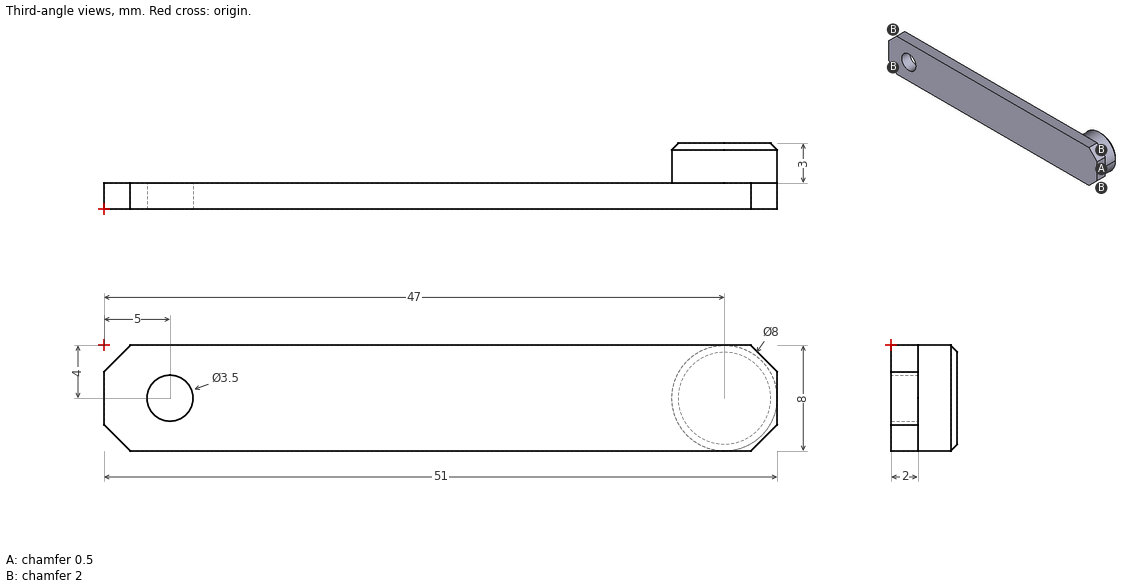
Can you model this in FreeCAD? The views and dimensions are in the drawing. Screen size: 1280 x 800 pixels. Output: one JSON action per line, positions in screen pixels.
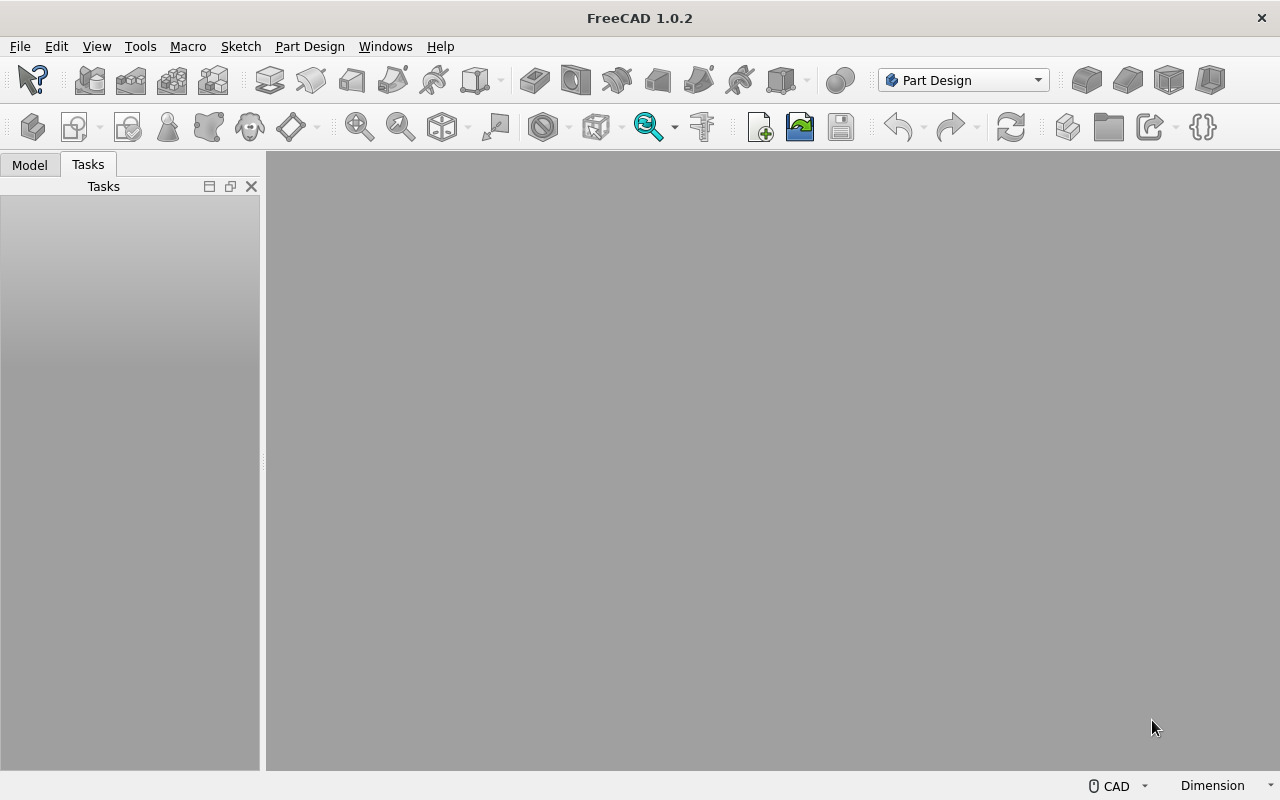
{"action": "key", "text": "ctrl+n"}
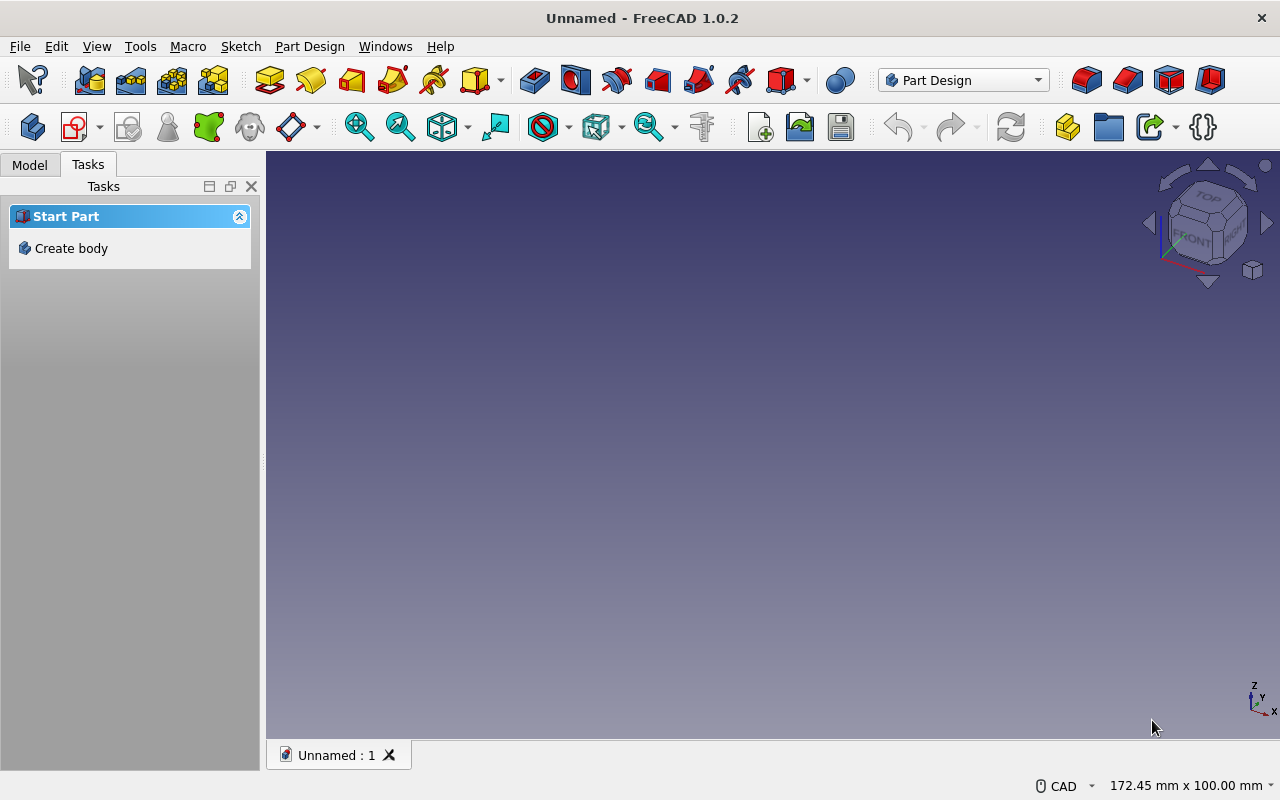
{"action": "left_click", "coordinate": [74, 128]}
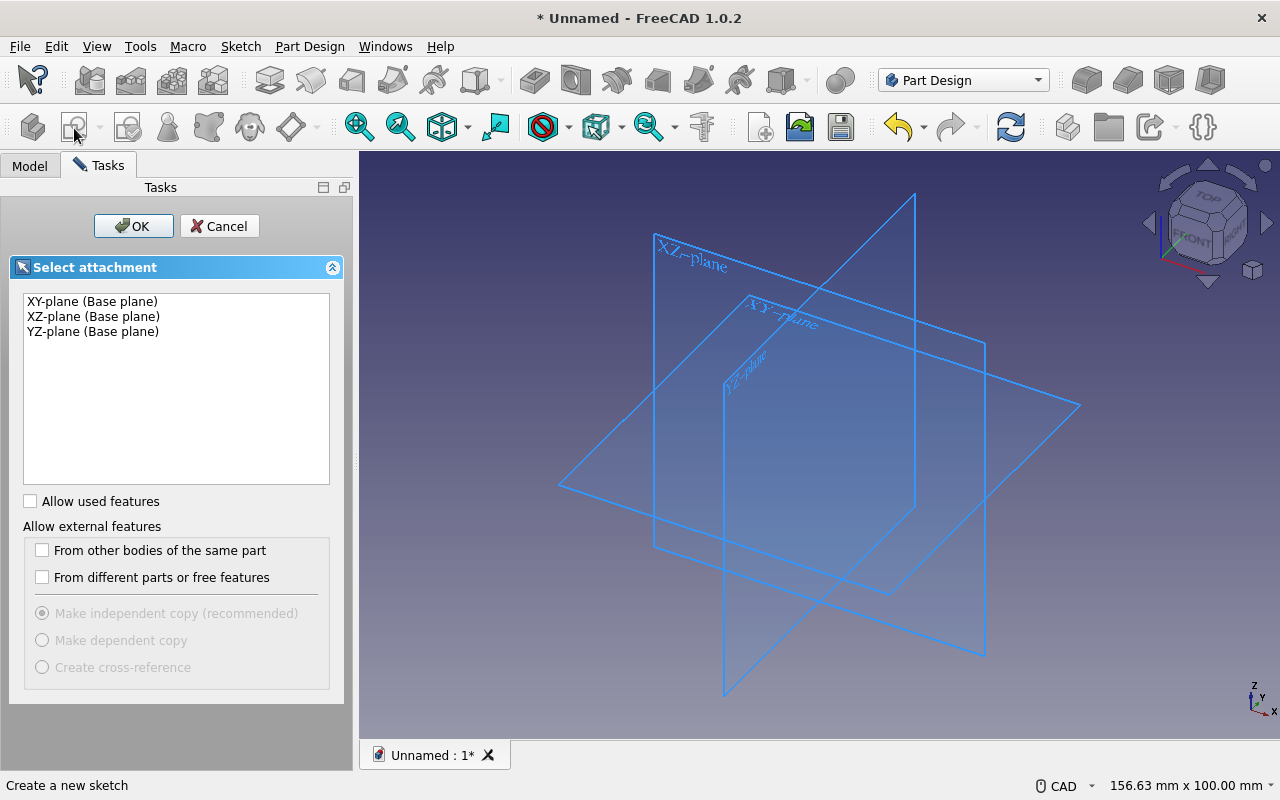
{"action": "left_click", "coordinate": [84, 316]}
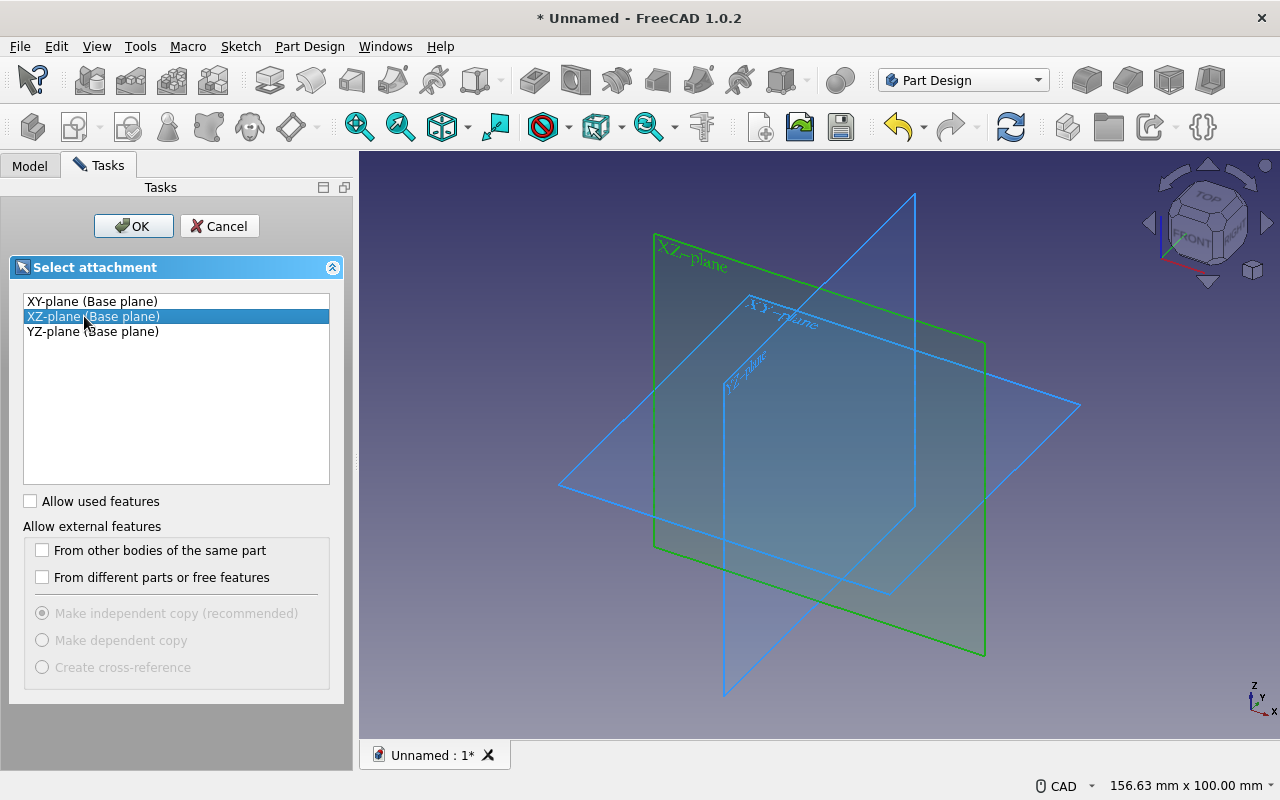
{"action": "left_click", "coordinate": [134, 226]}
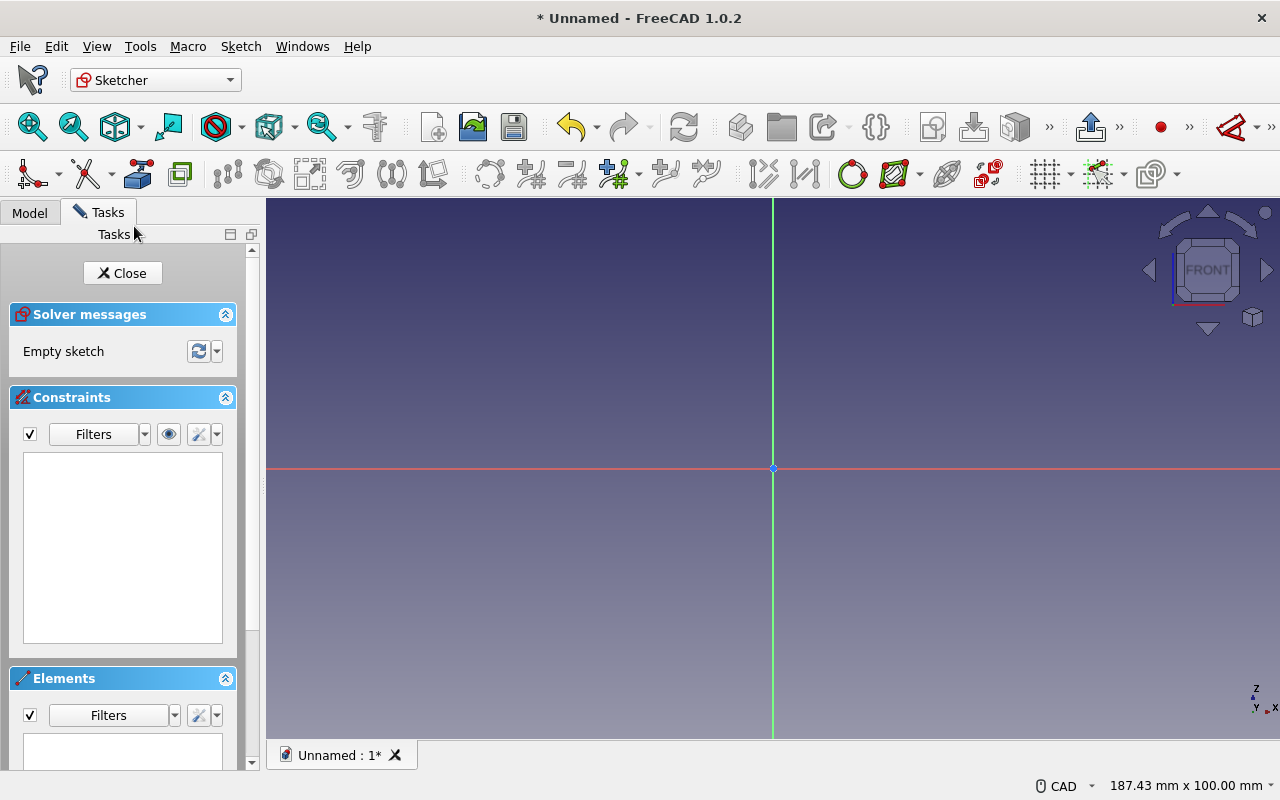
{"action": "scroll", "coordinate": [1079, 508], "scroll_direction": "up", "scroll_amount": 4}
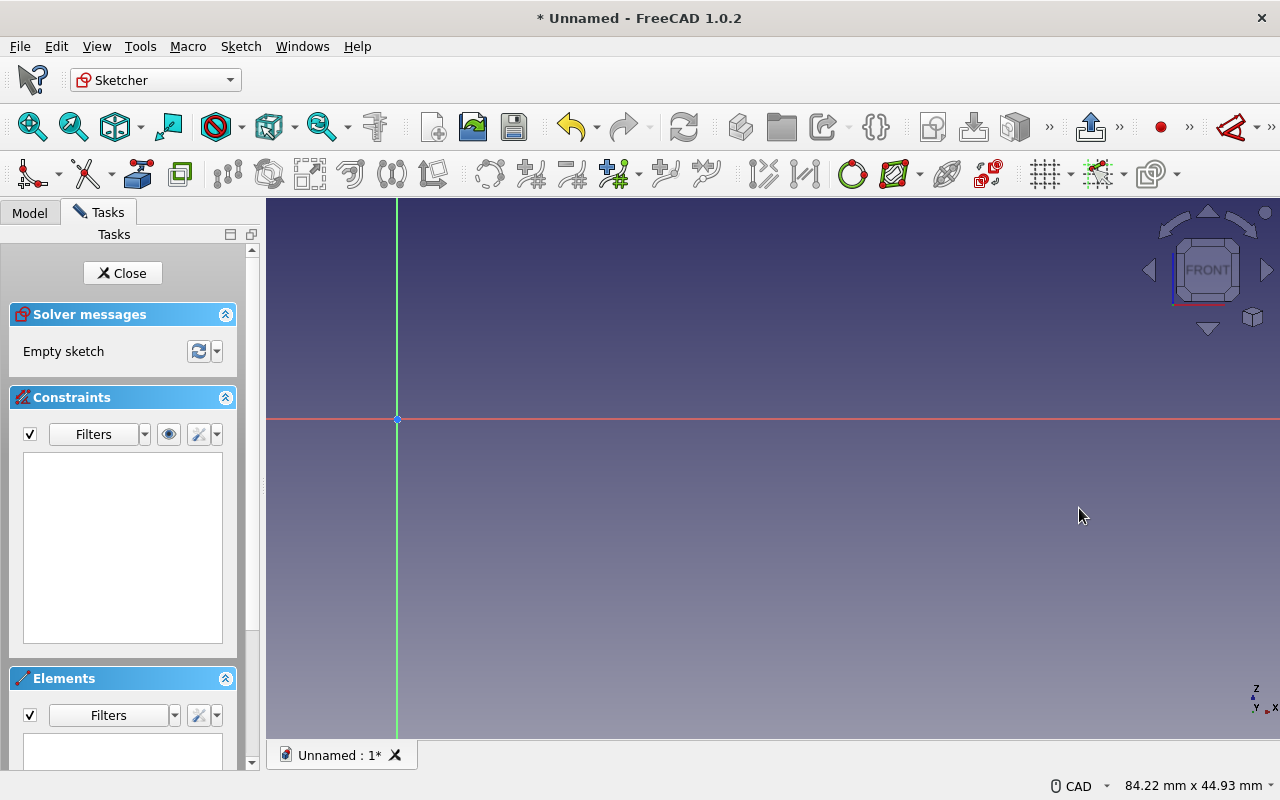
{"action": "key", "text": "g r"}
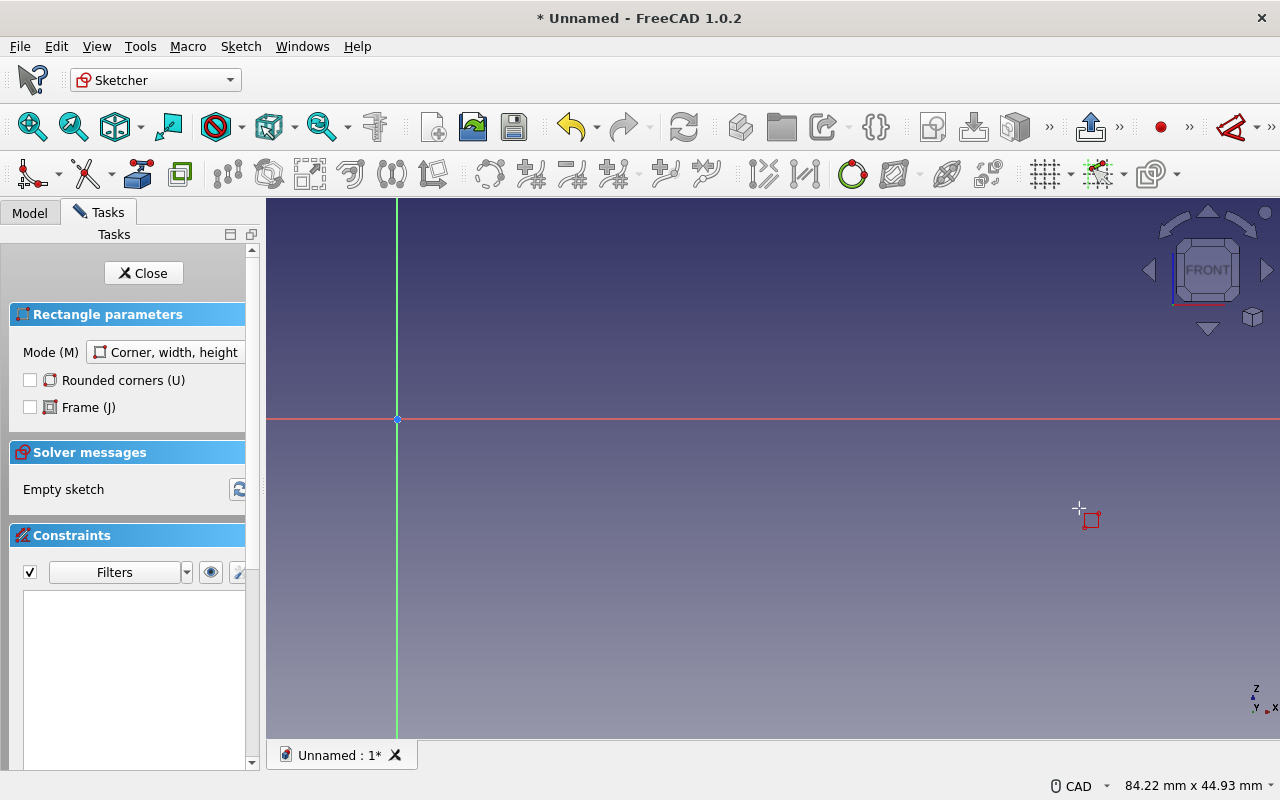
{"action": "left_click", "coordinate": [397, 419]}
{"action": "mouse_move", "coordinate": [1011, 516]}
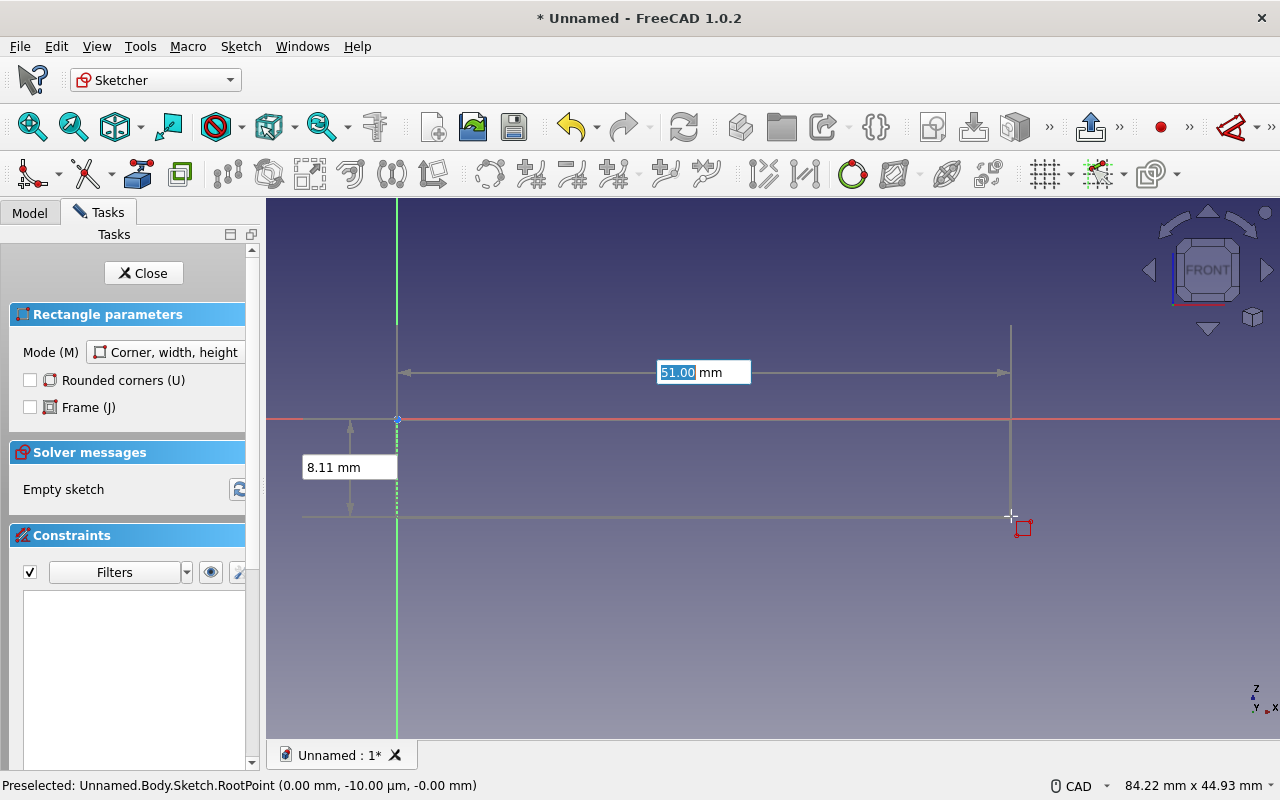
{"action": "type", "text": "51"}
{"action": "key", "text": "Tab"}
{"action": "type", "text": "8"}
{"action": "key", "text": "Return"}
{"action": "key", "text": "Escape"}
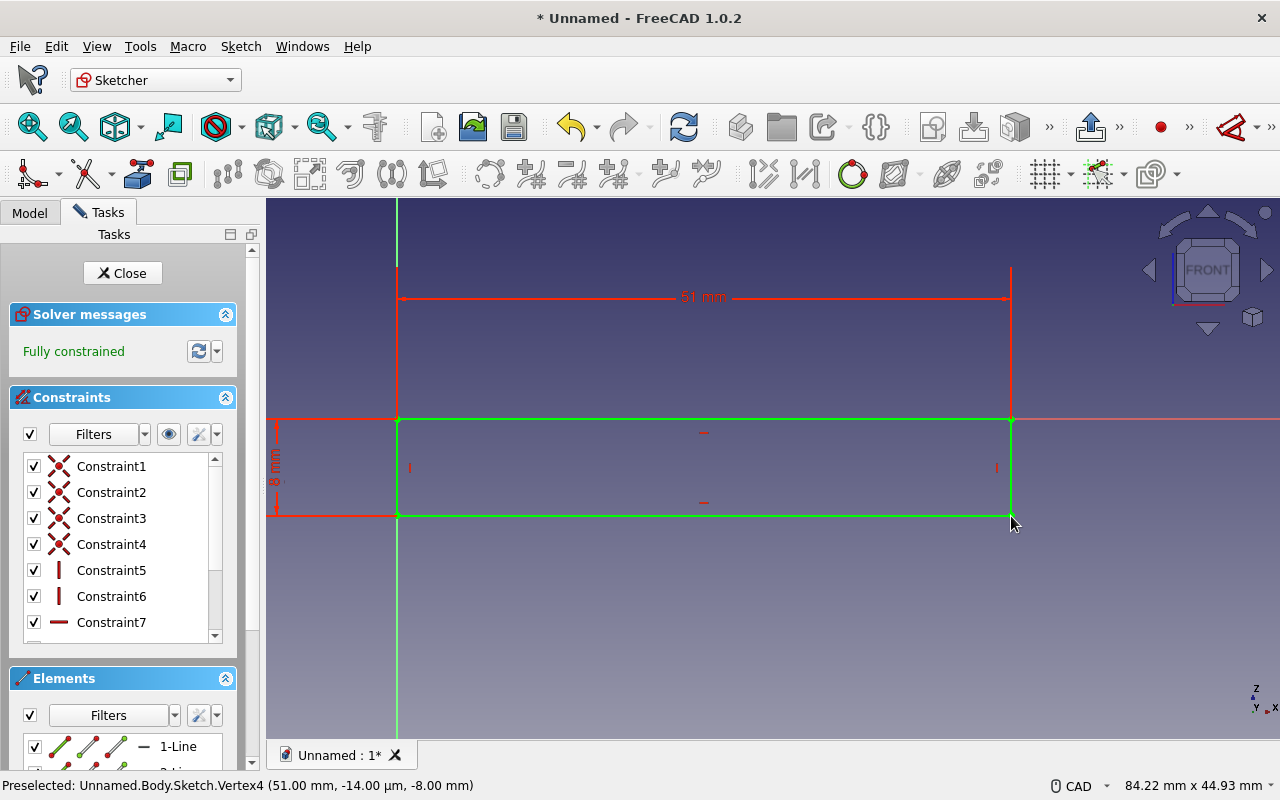
{"action": "left_click", "coordinate": [123, 273]}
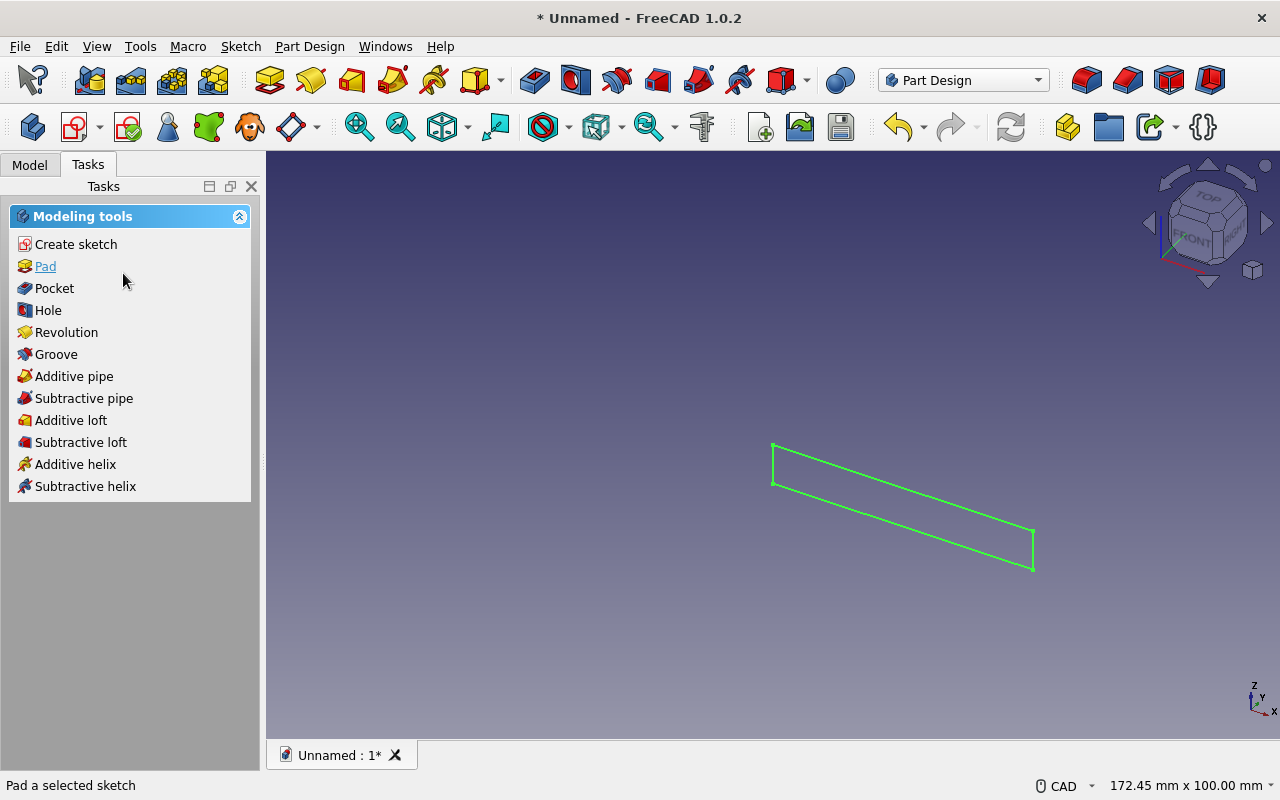
{"action": "left_click", "coordinate": [270, 80]}